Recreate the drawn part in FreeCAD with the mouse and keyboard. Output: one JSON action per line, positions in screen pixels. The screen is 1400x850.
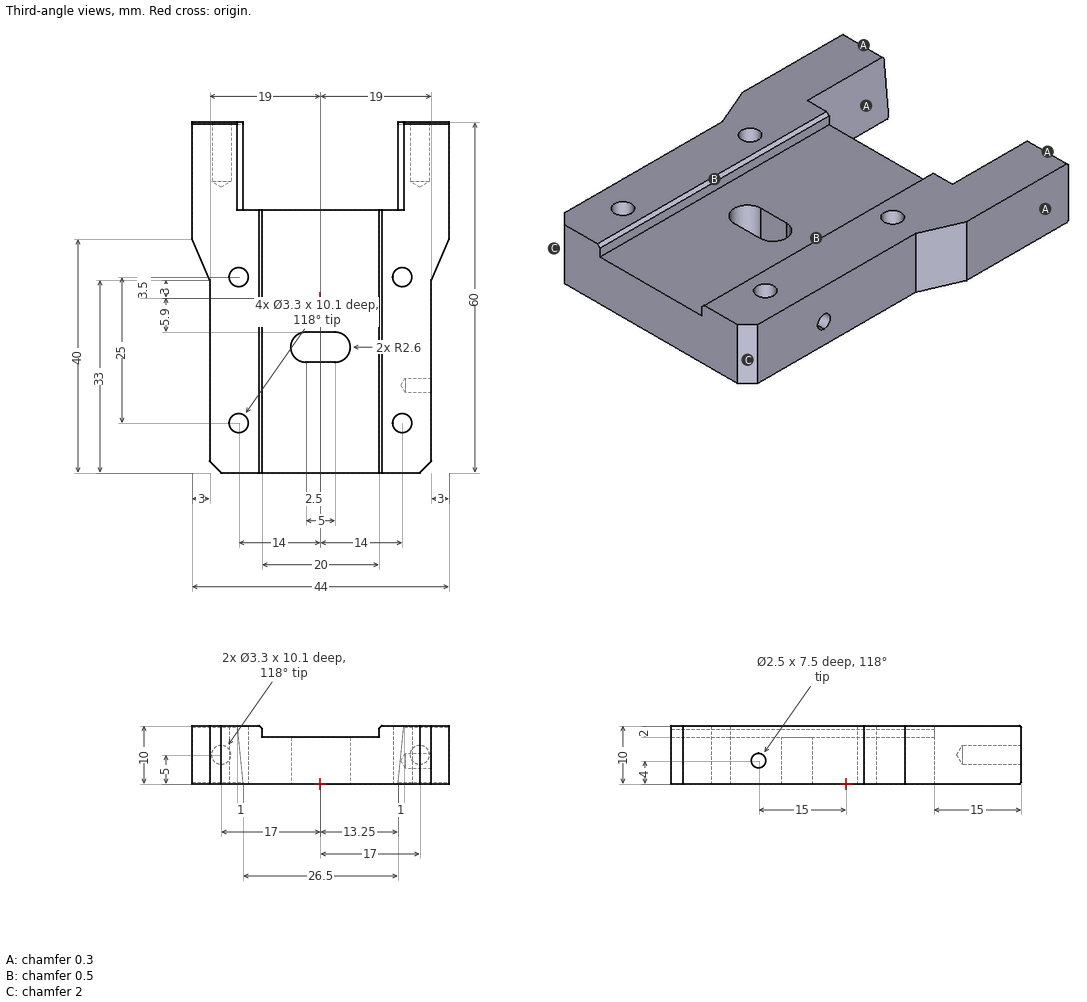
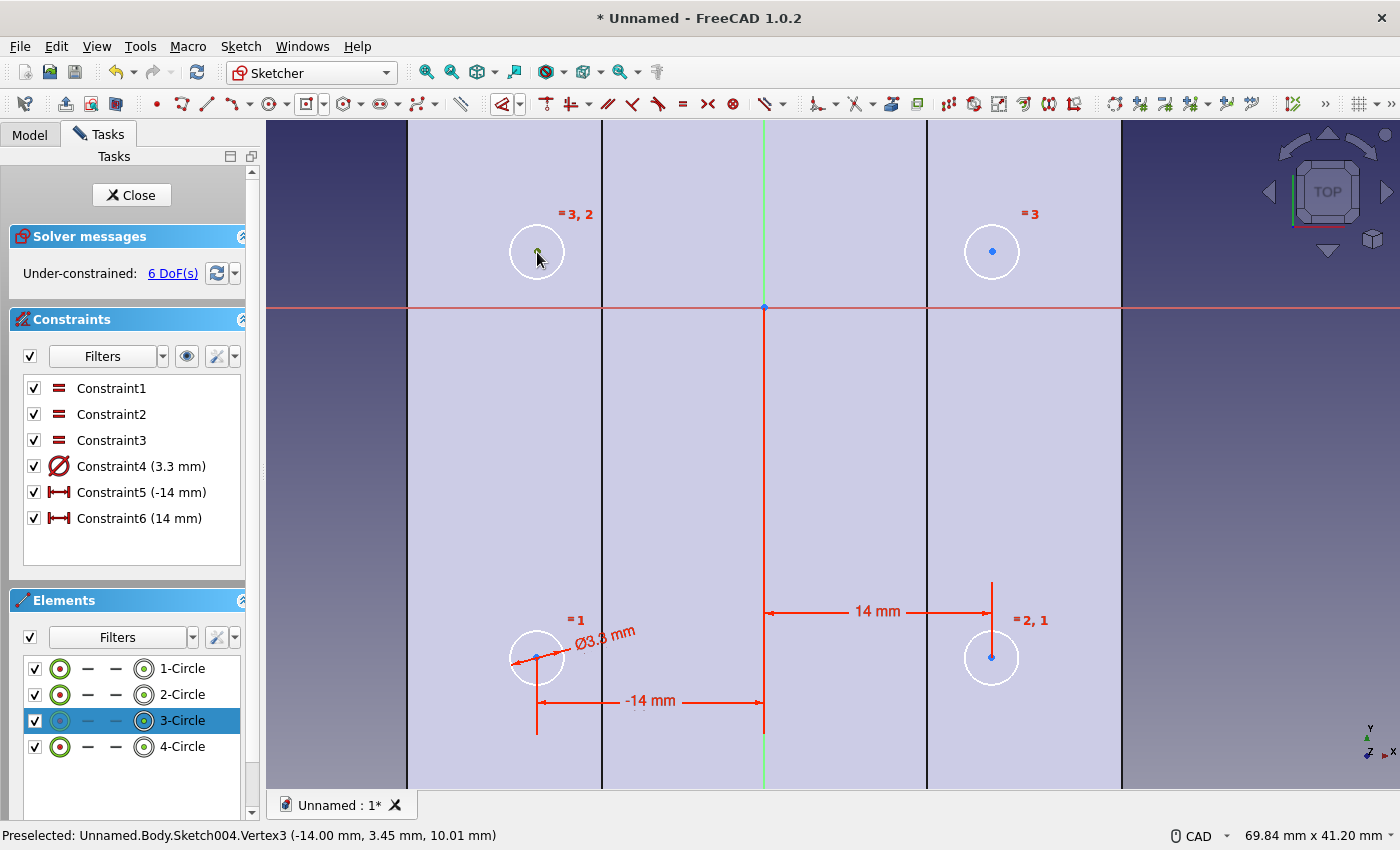
{"action": "key", "text": "l"}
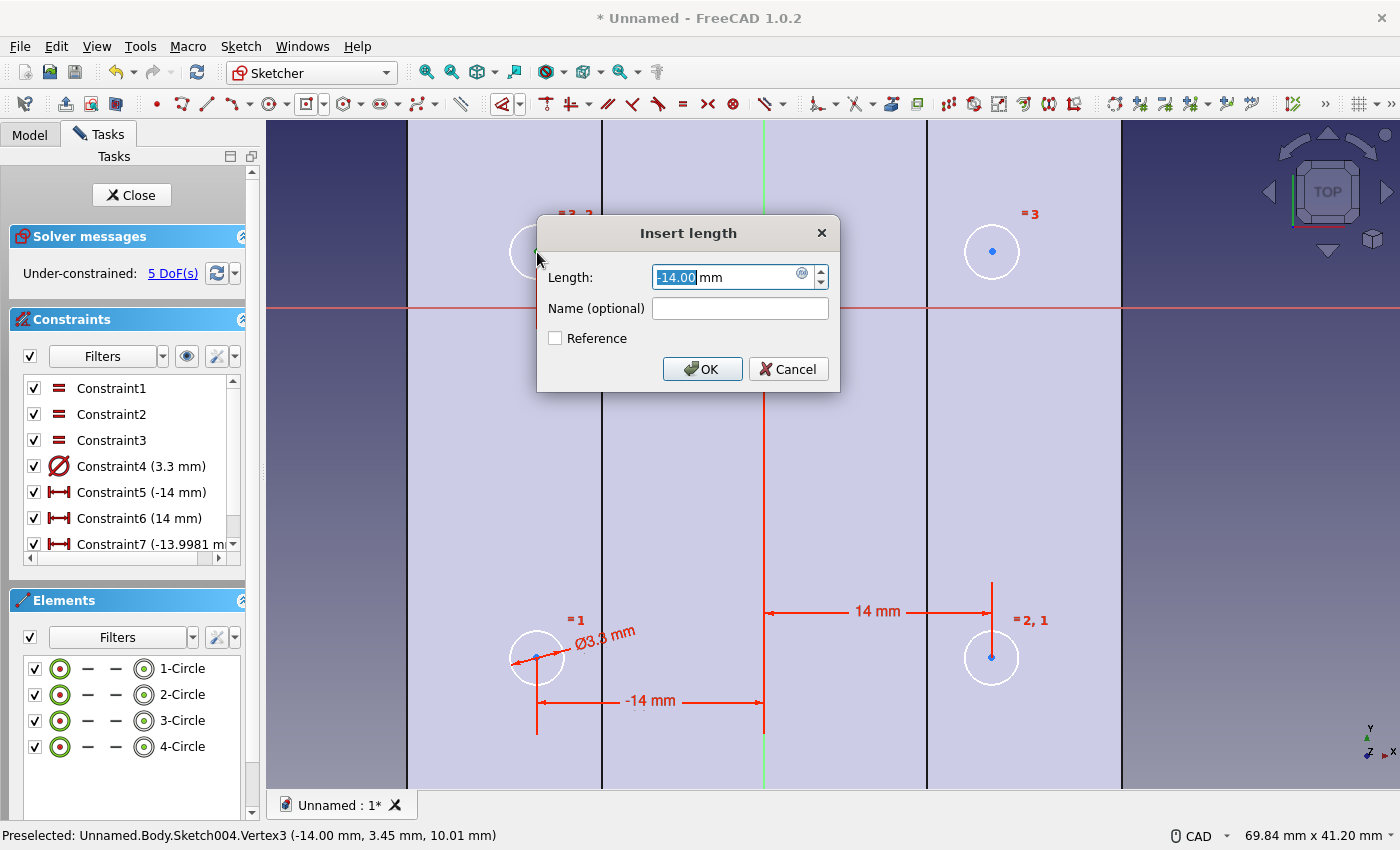
{"action": "type", "text": "-14"}
{"action": "key", "text": "Return"}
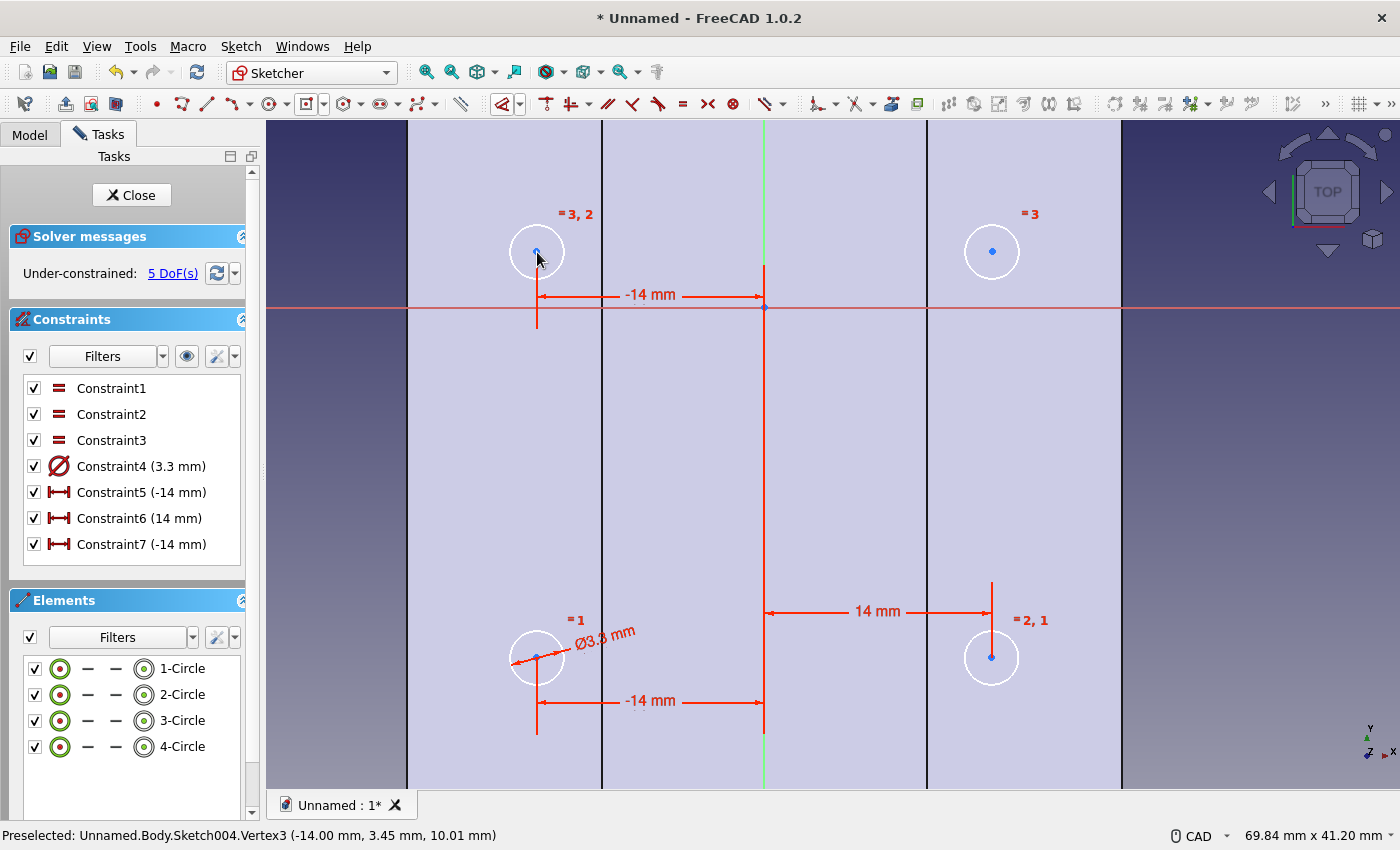
{"action": "left_click", "coordinate": [992, 252]}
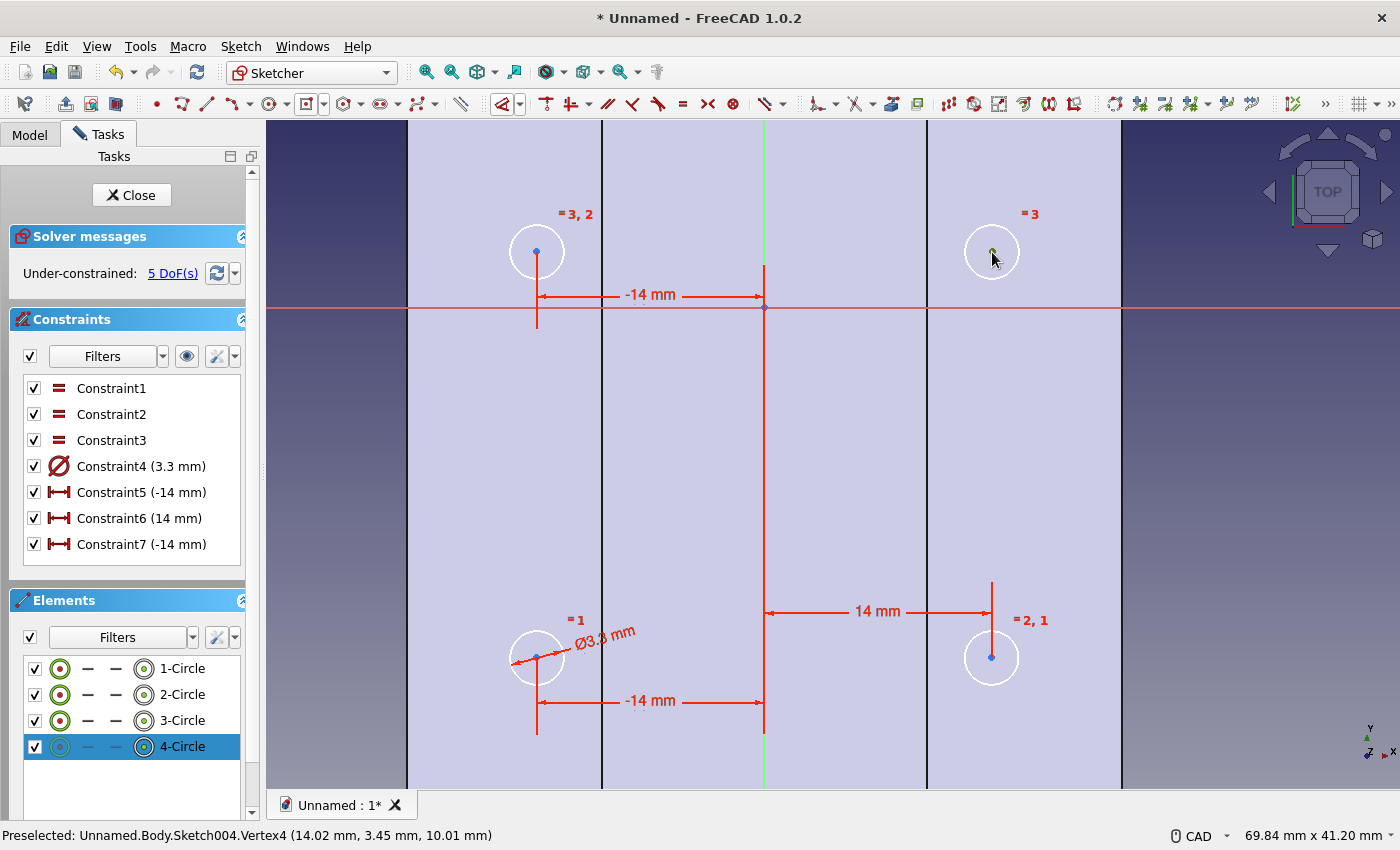
{"action": "key", "text": "l"}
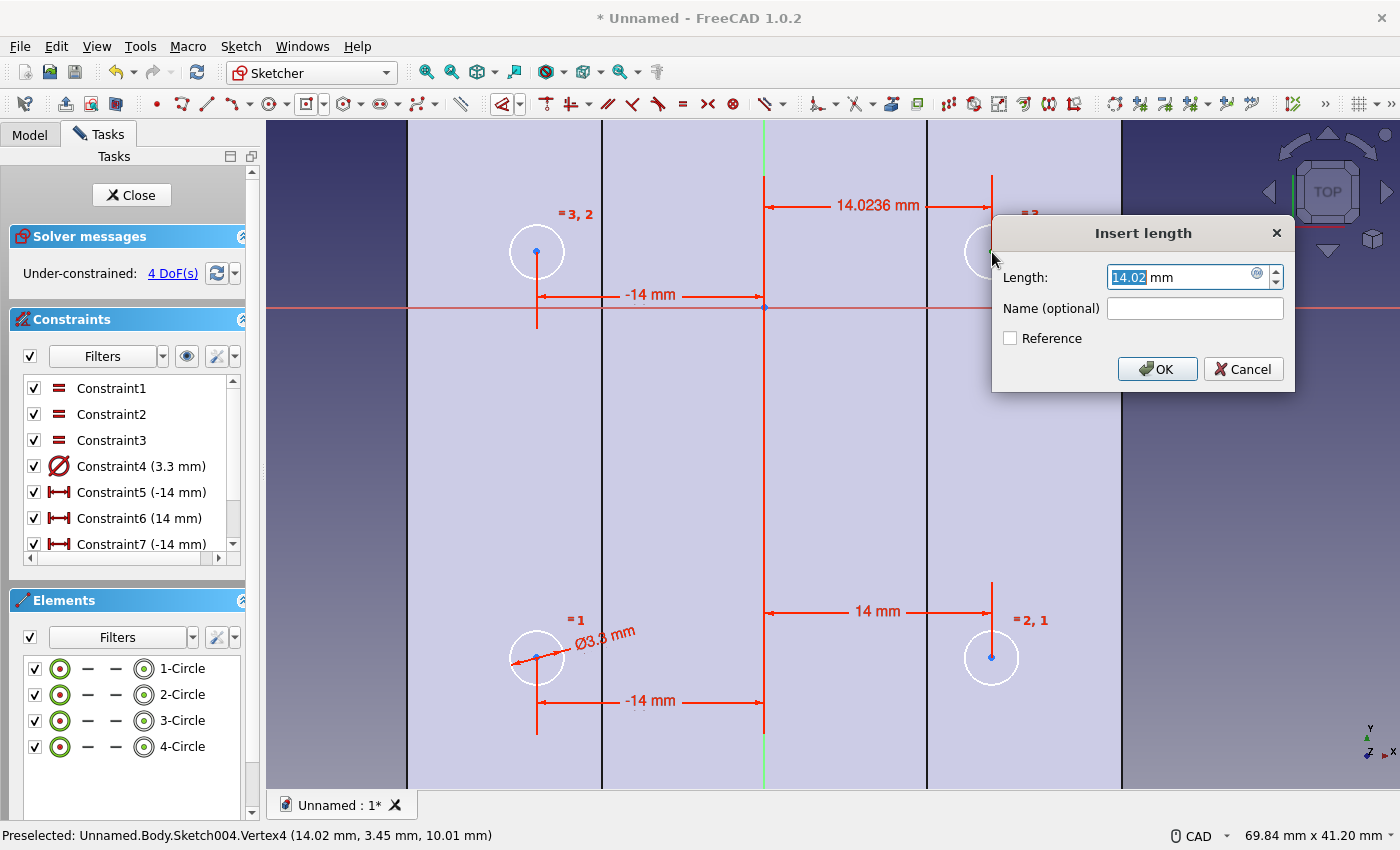
{"action": "type", "text": "14"}
{"action": "key", "text": "Return"}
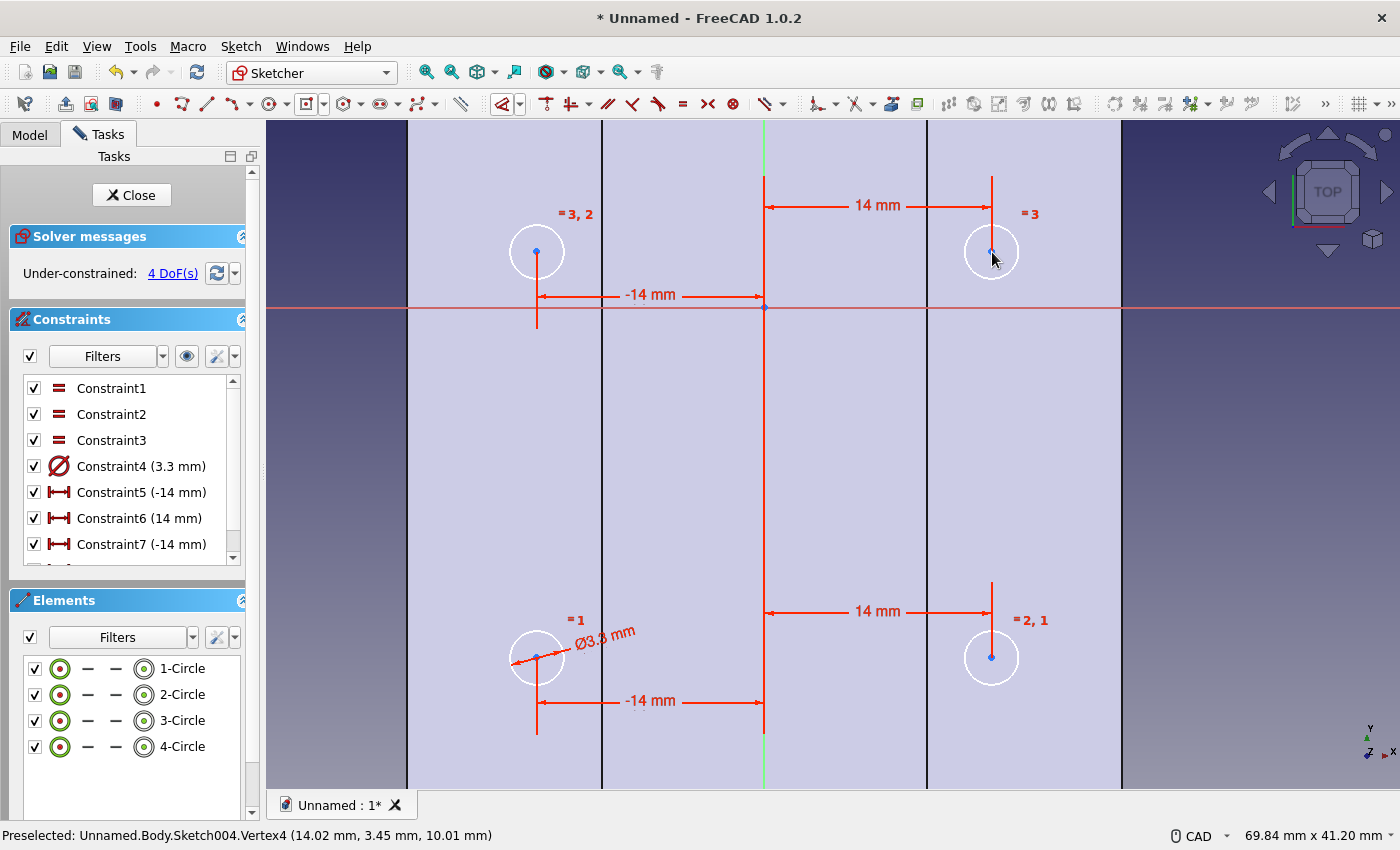
{"action": "left_click", "coordinate": [537, 252]}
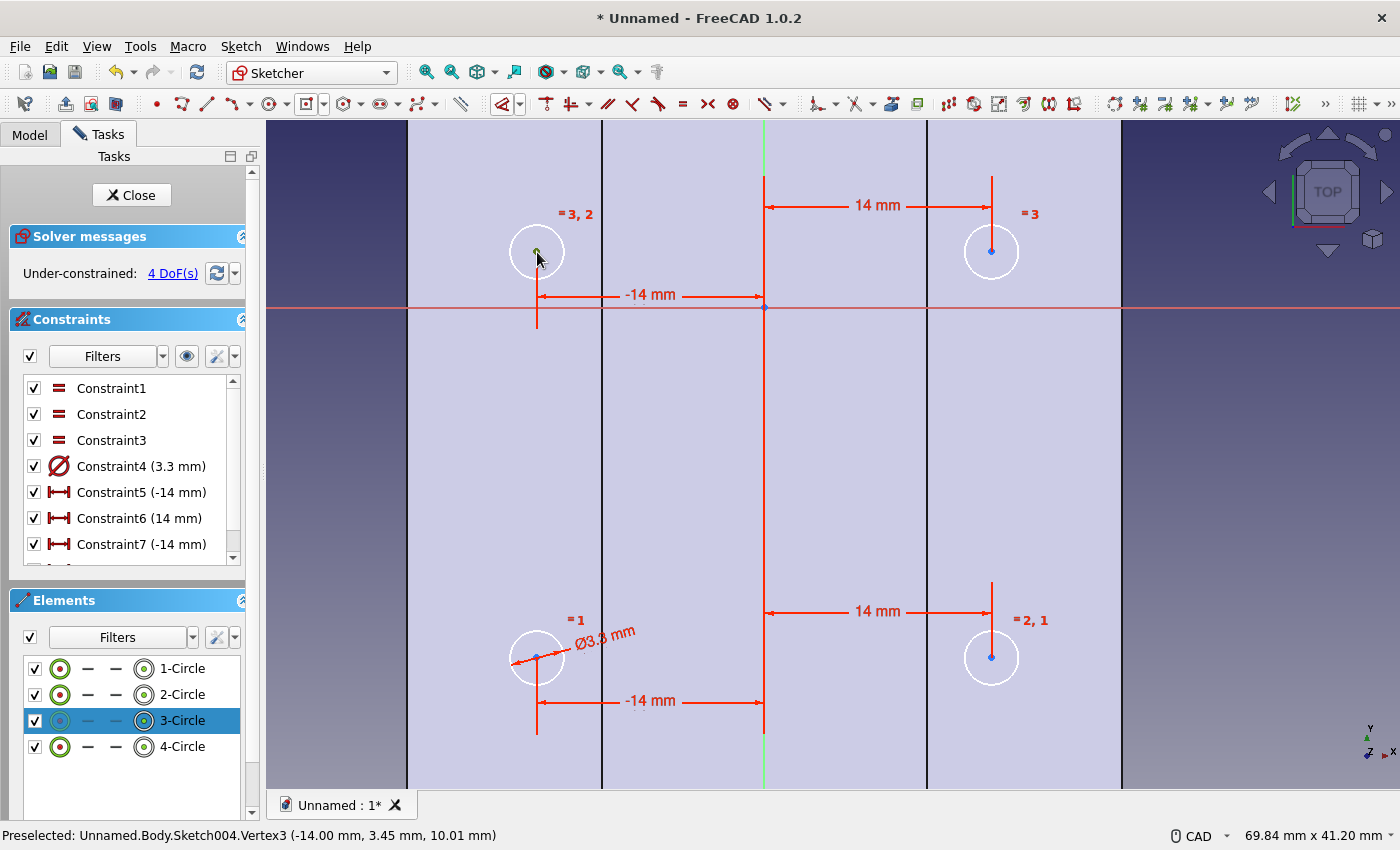
{"action": "left_click", "coordinate": [520, 104]}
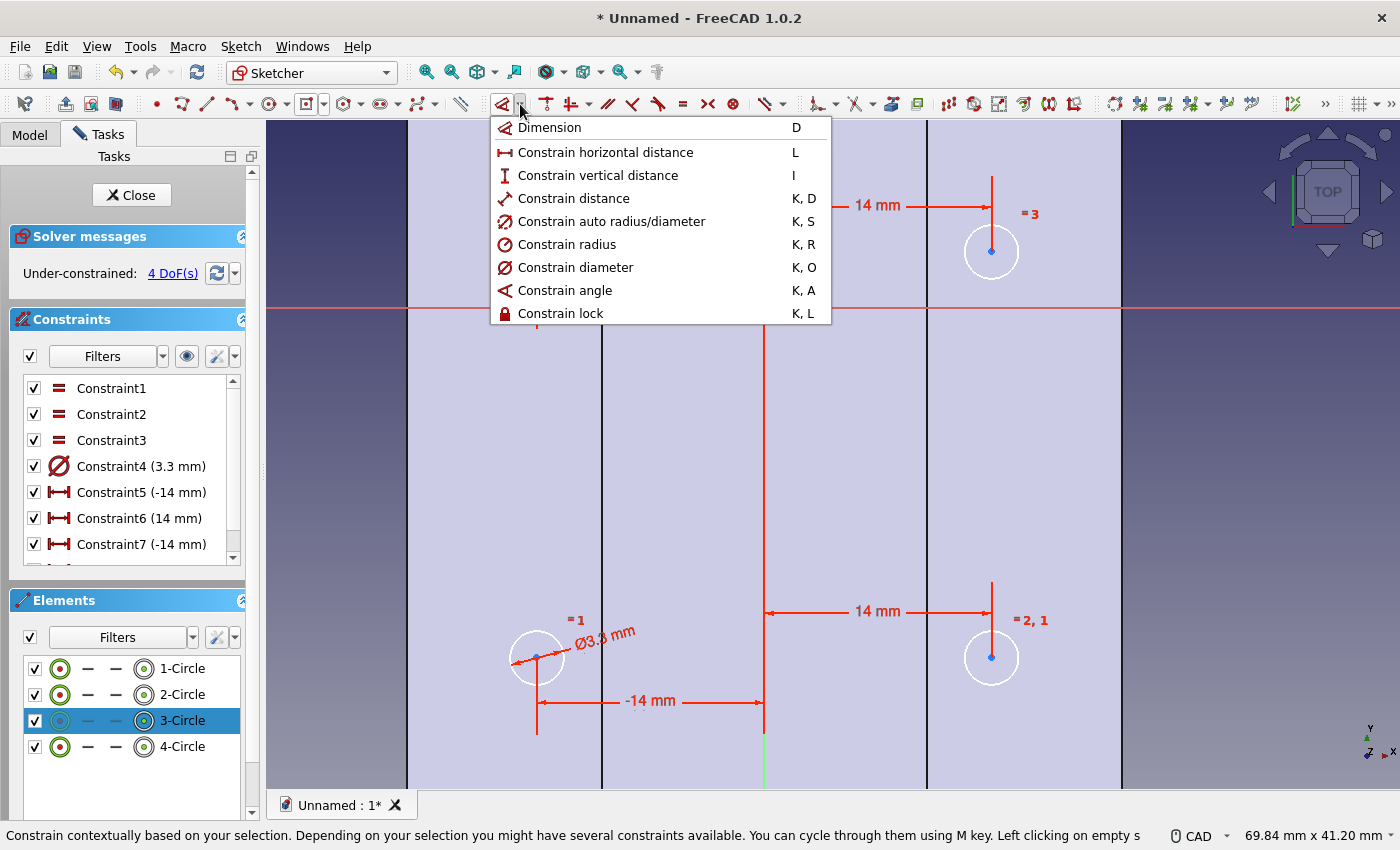
{"action": "left_click", "coordinate": [661, 176]}